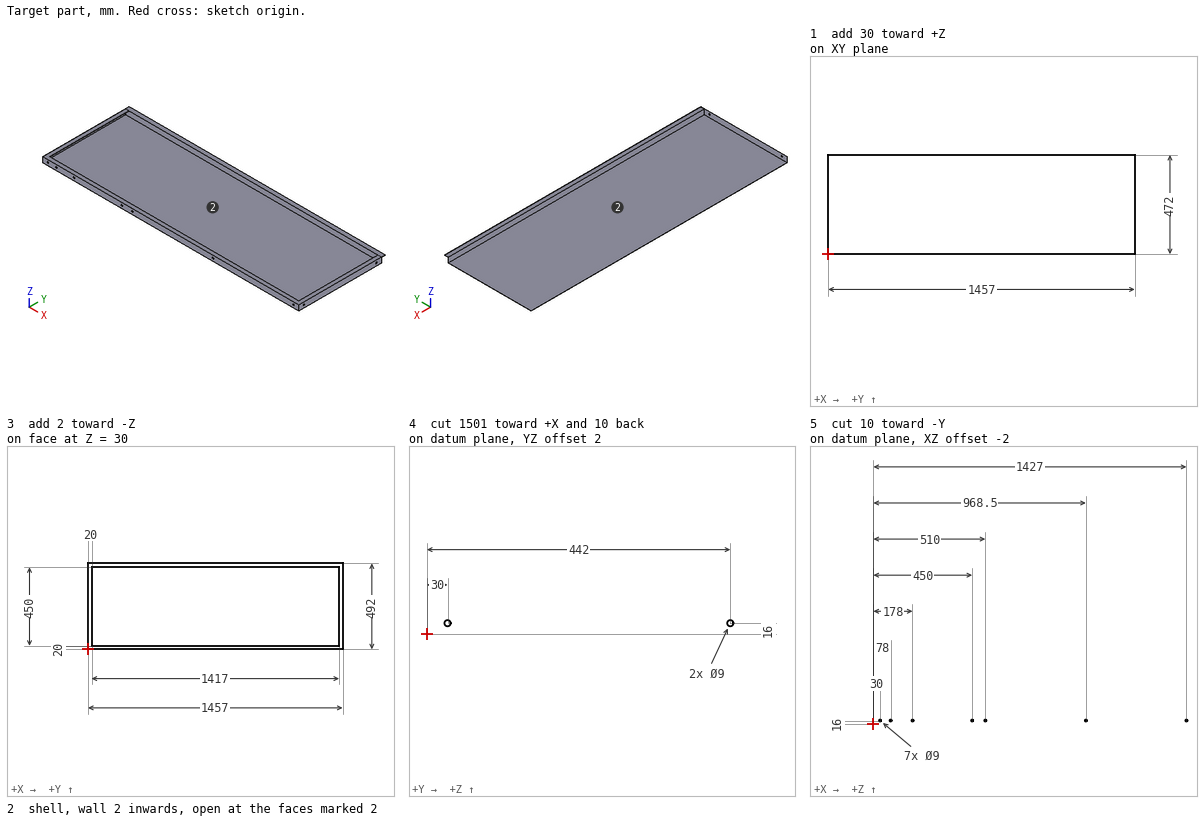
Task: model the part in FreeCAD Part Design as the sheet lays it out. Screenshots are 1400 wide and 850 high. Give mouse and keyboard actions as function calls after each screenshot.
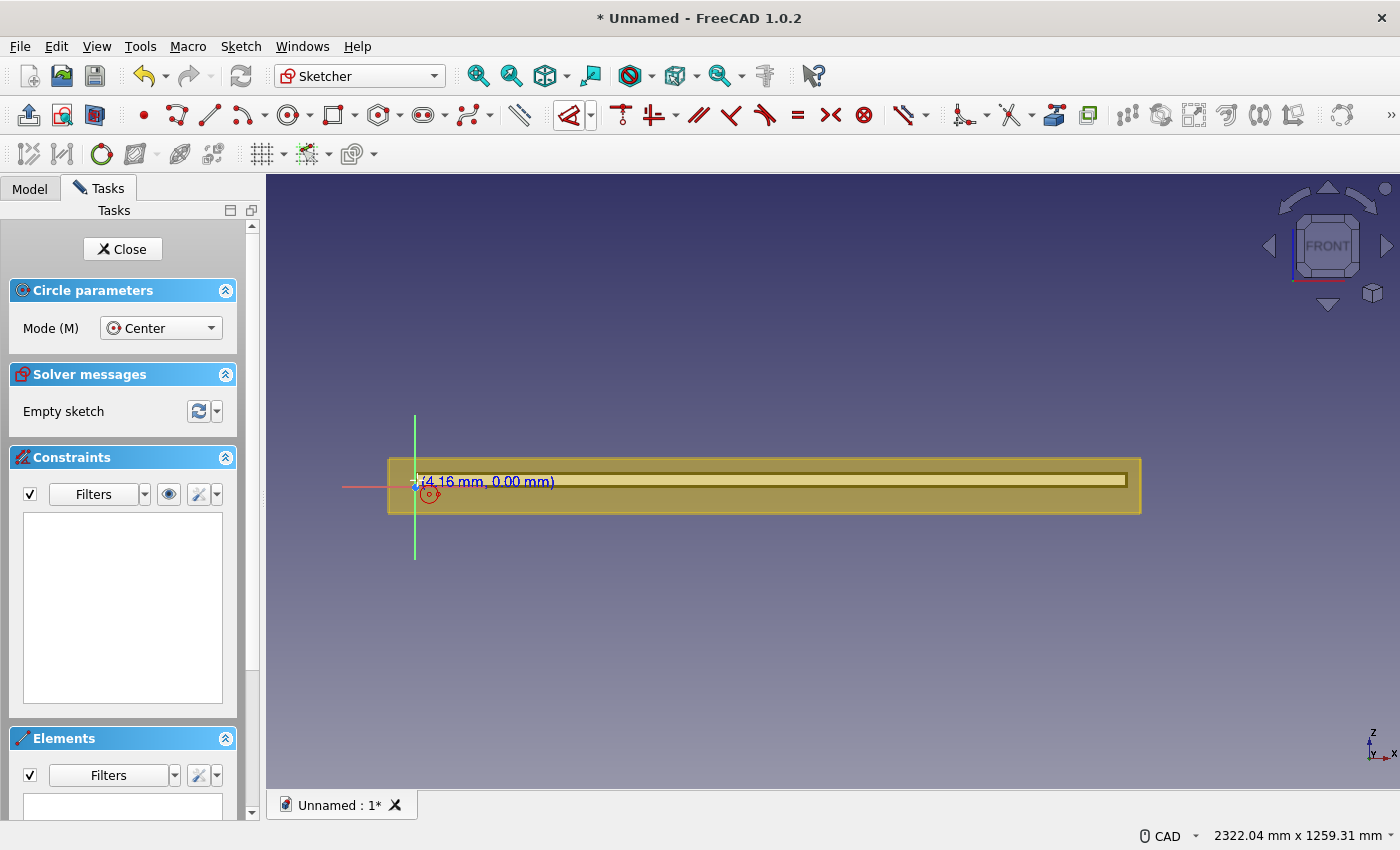
scroll(430, 479, up, 4)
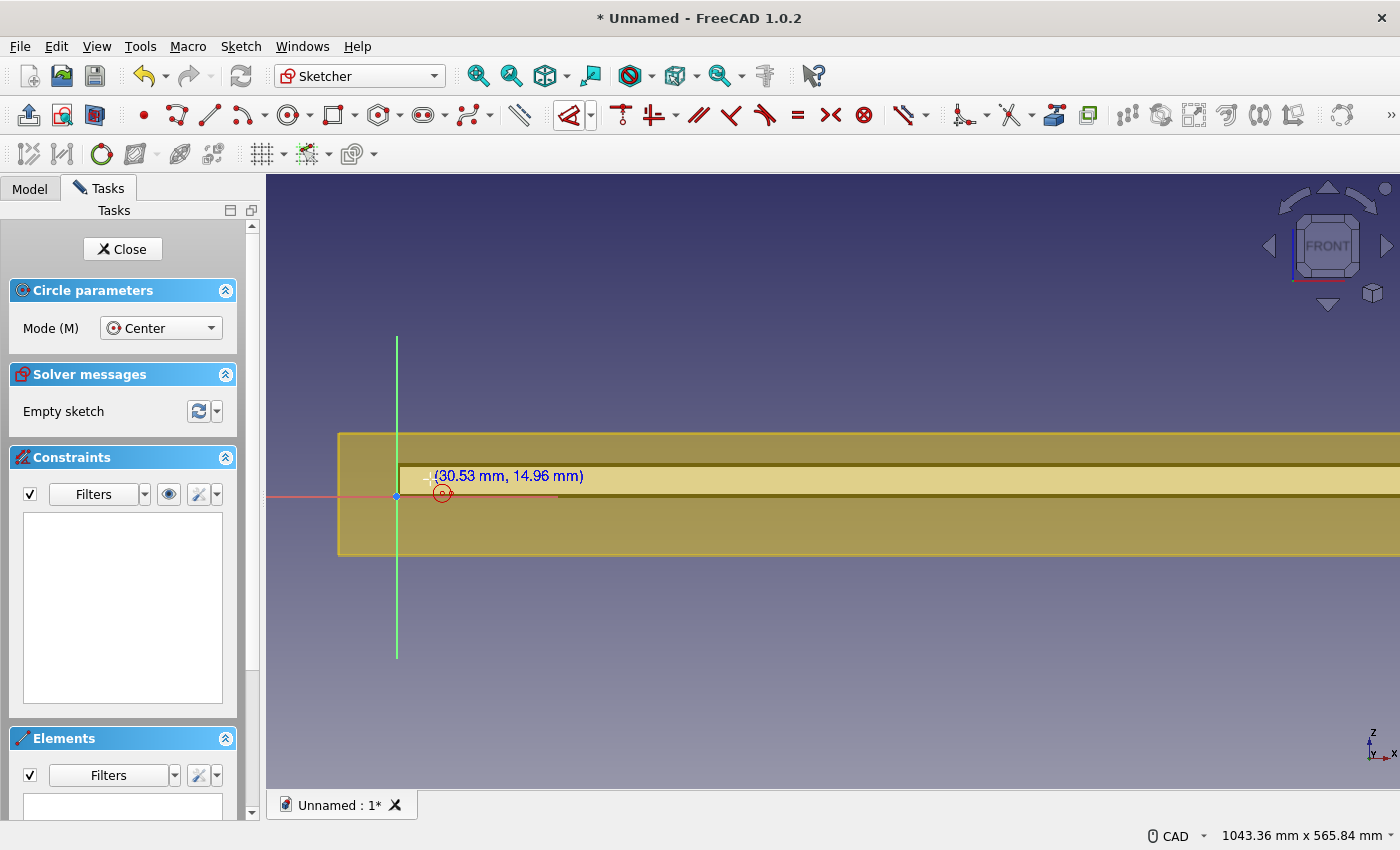
click(429, 479)
move(433, 476)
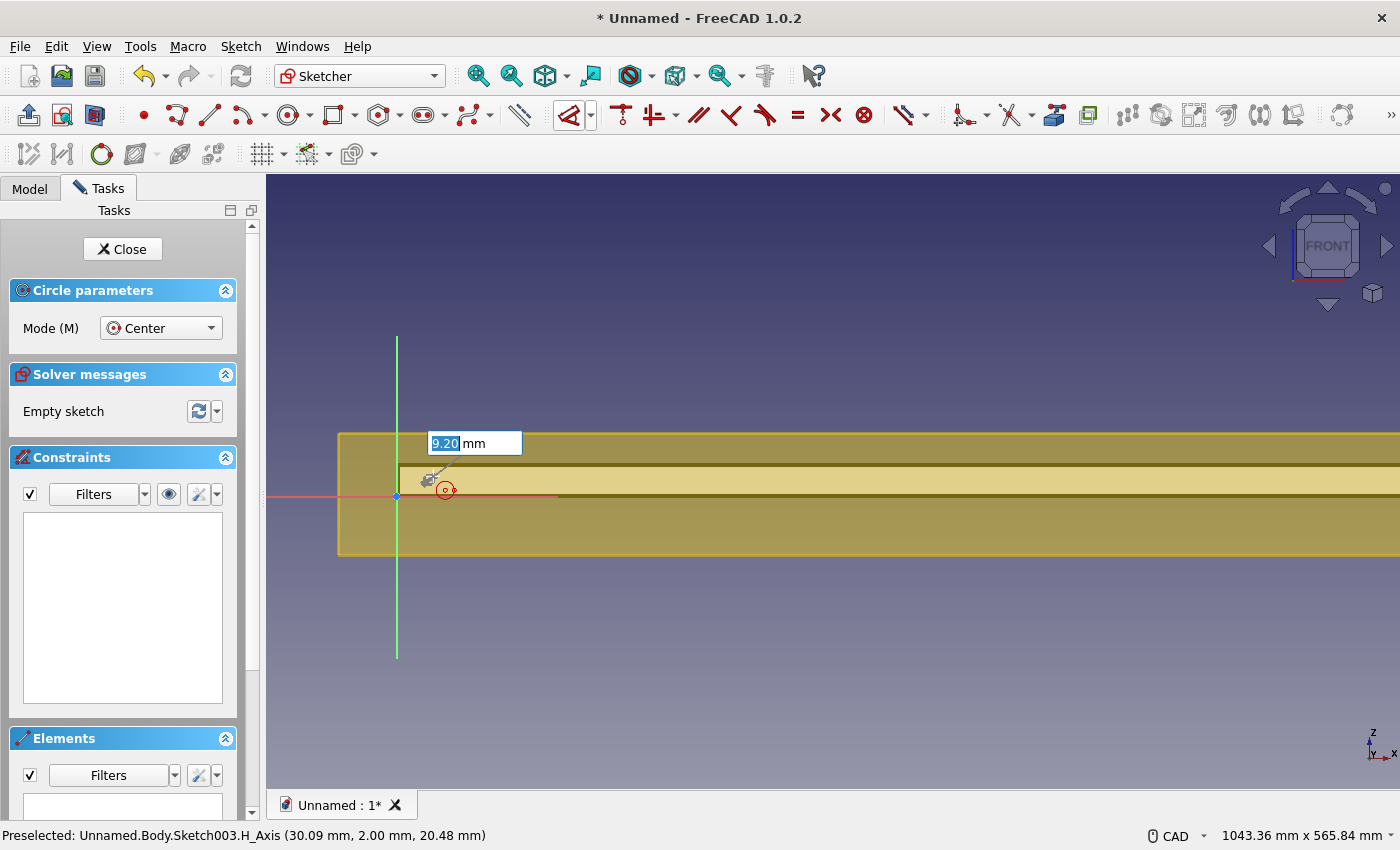
text(9)
key(Return)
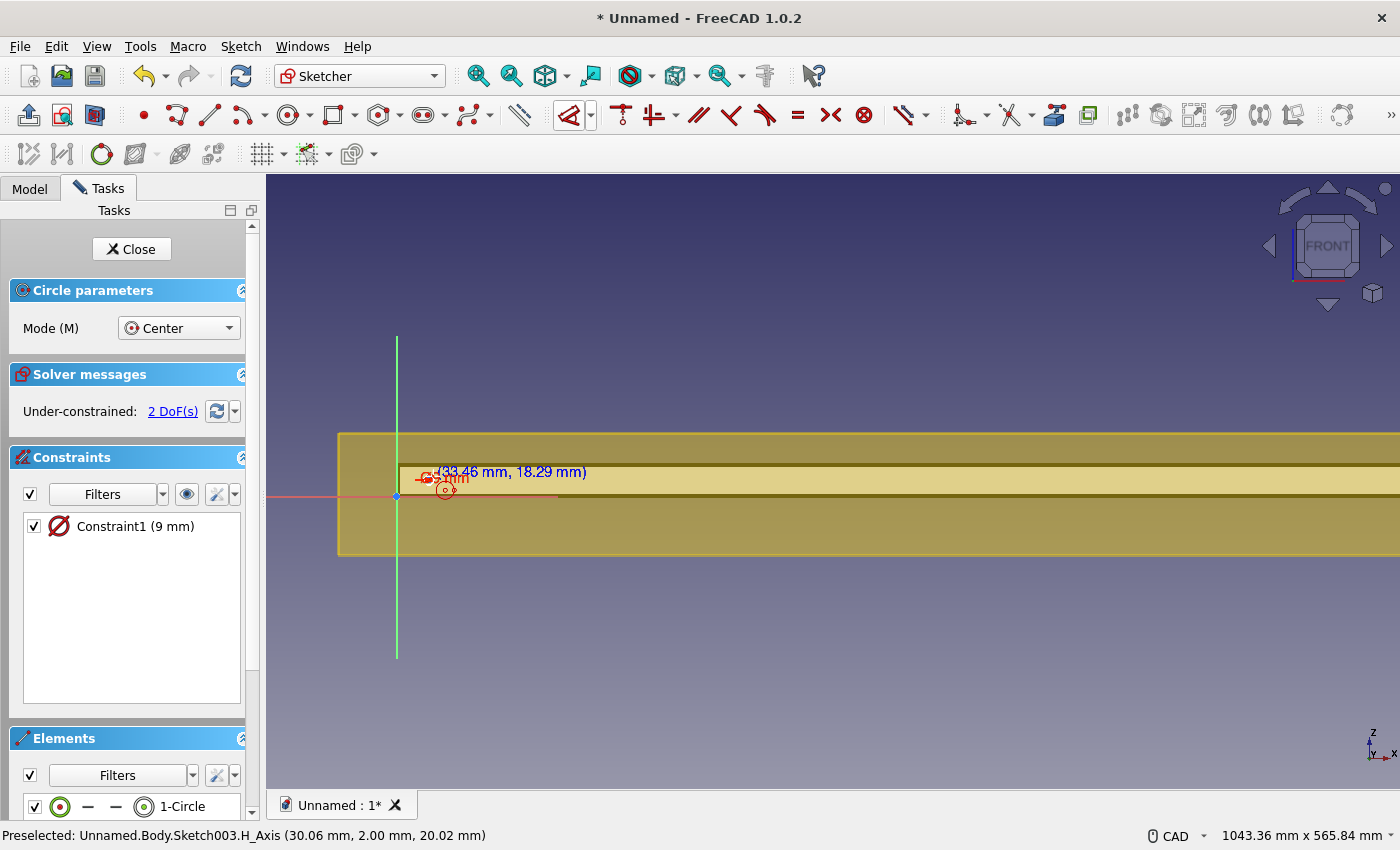
scroll(886, 479, up, 8)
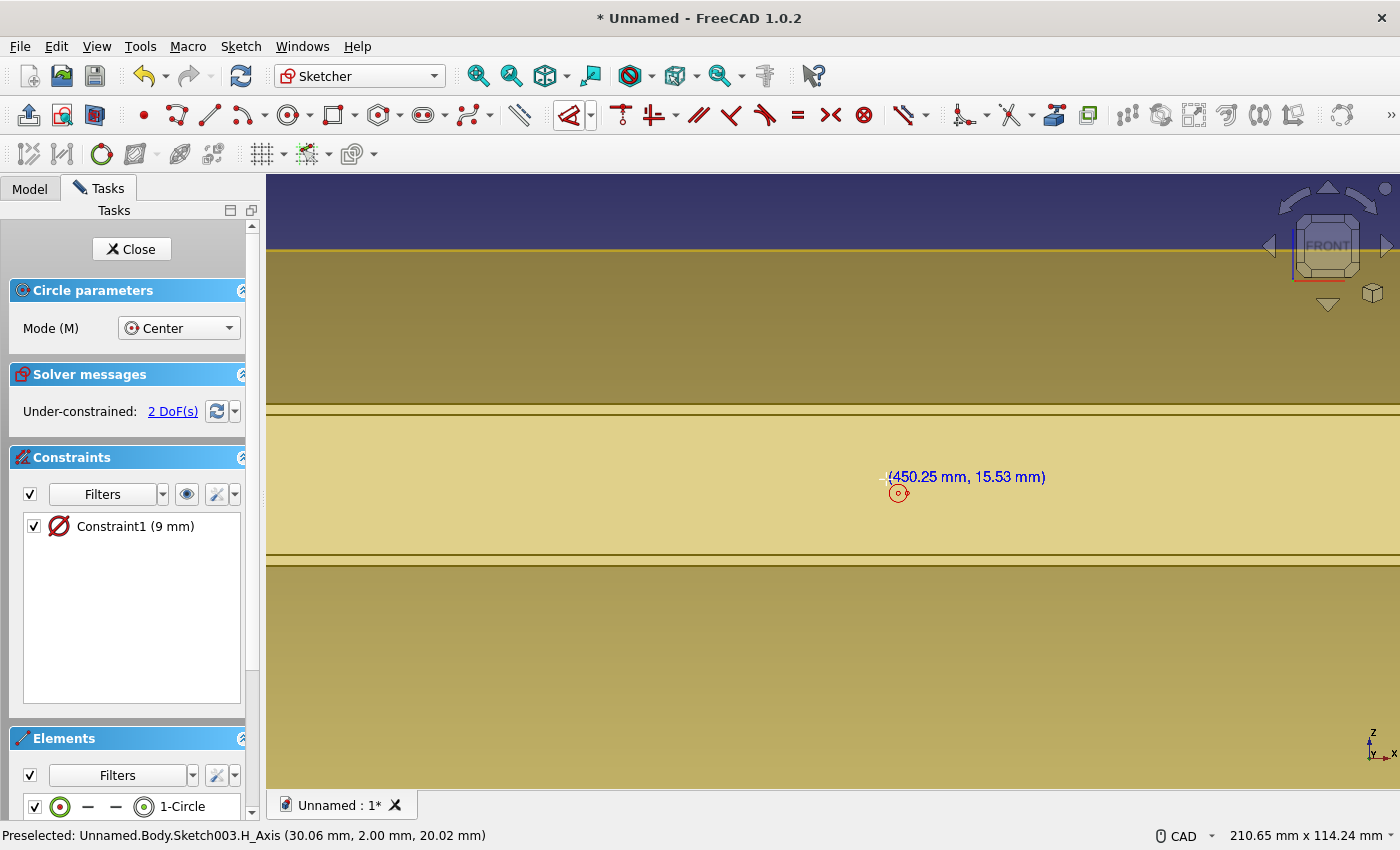
scroll(610, 479, down, 12)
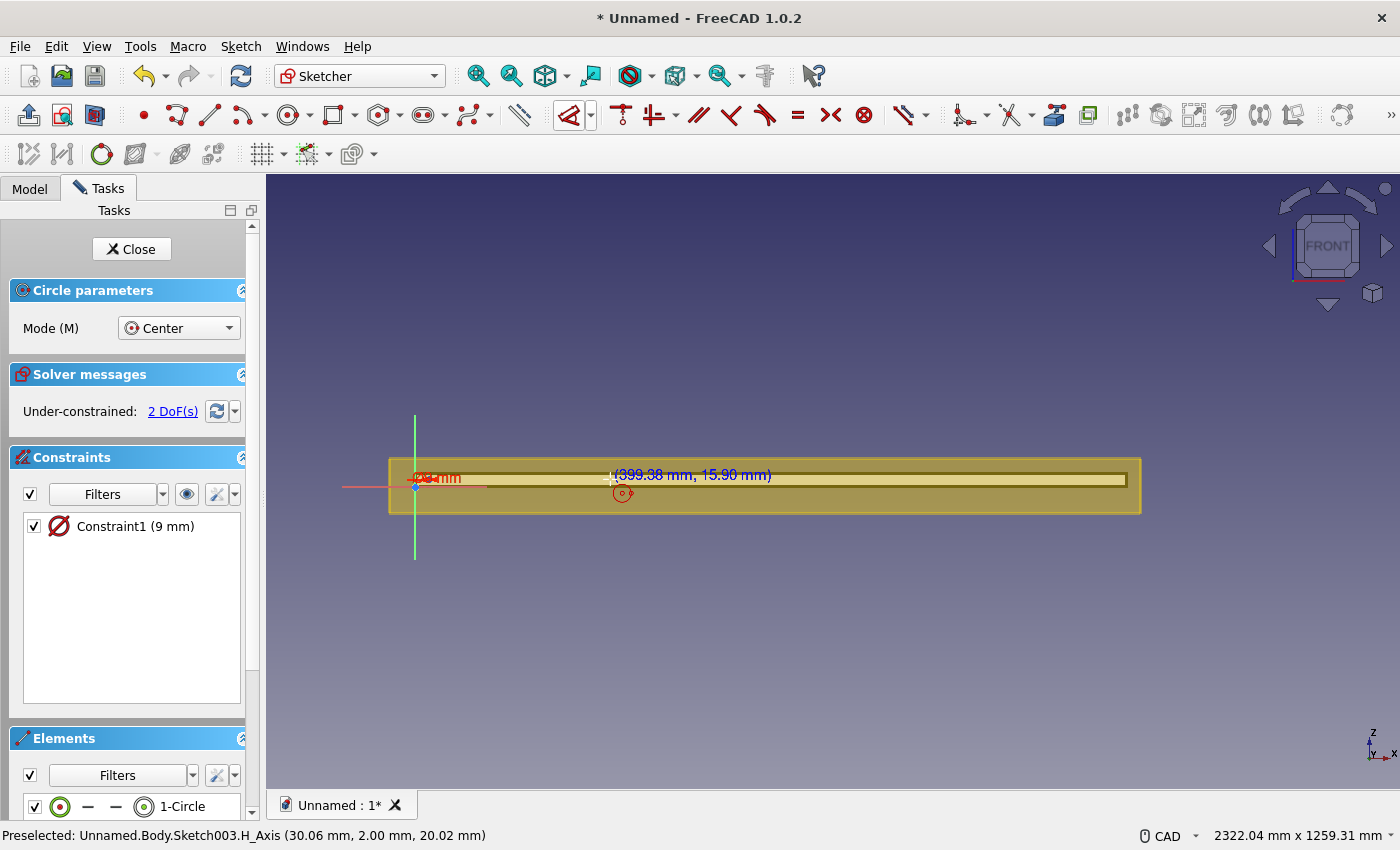
scroll(635, 479, up, 4)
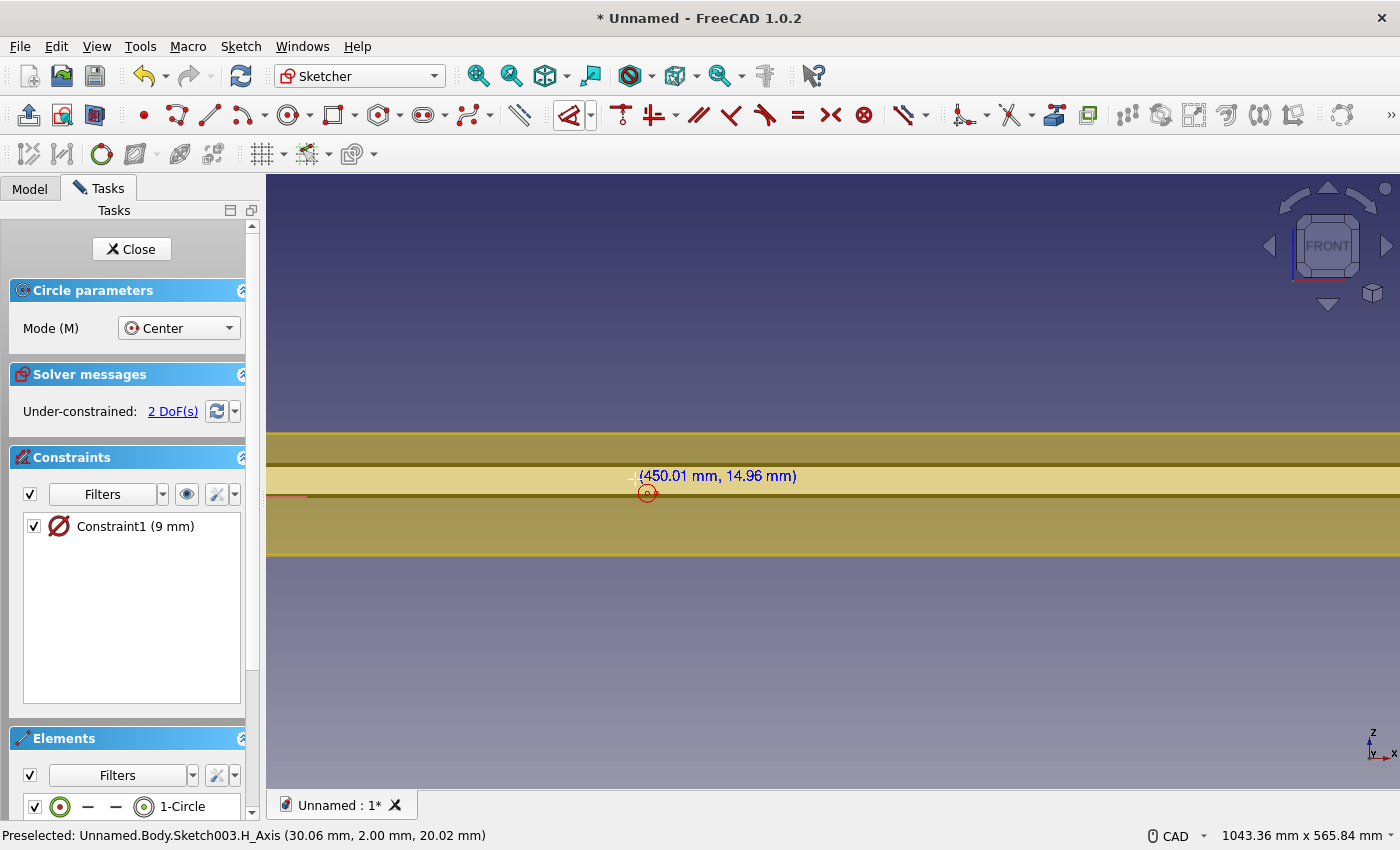
click(635, 479)
move(638, 476)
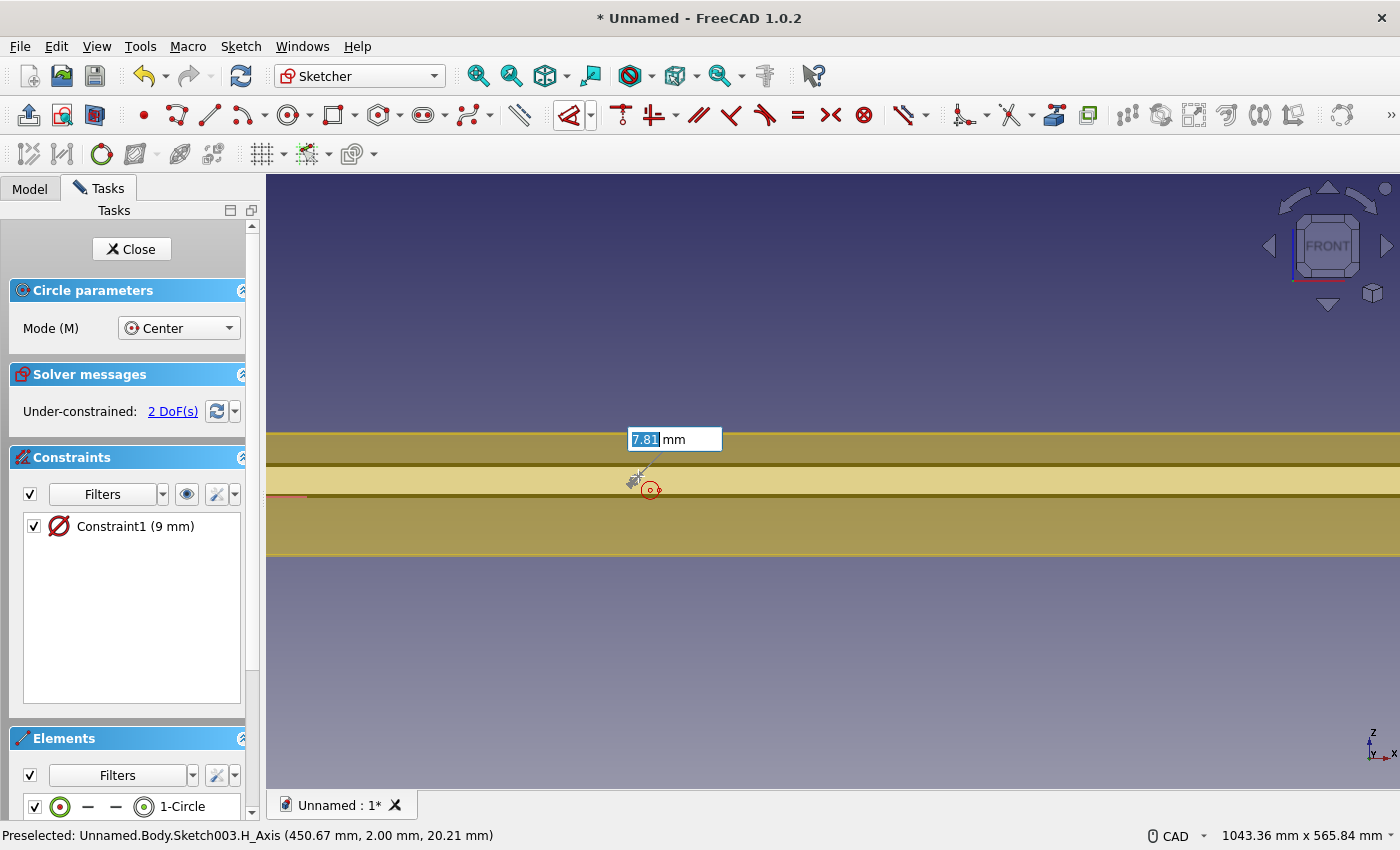
text(9)
key(Return)